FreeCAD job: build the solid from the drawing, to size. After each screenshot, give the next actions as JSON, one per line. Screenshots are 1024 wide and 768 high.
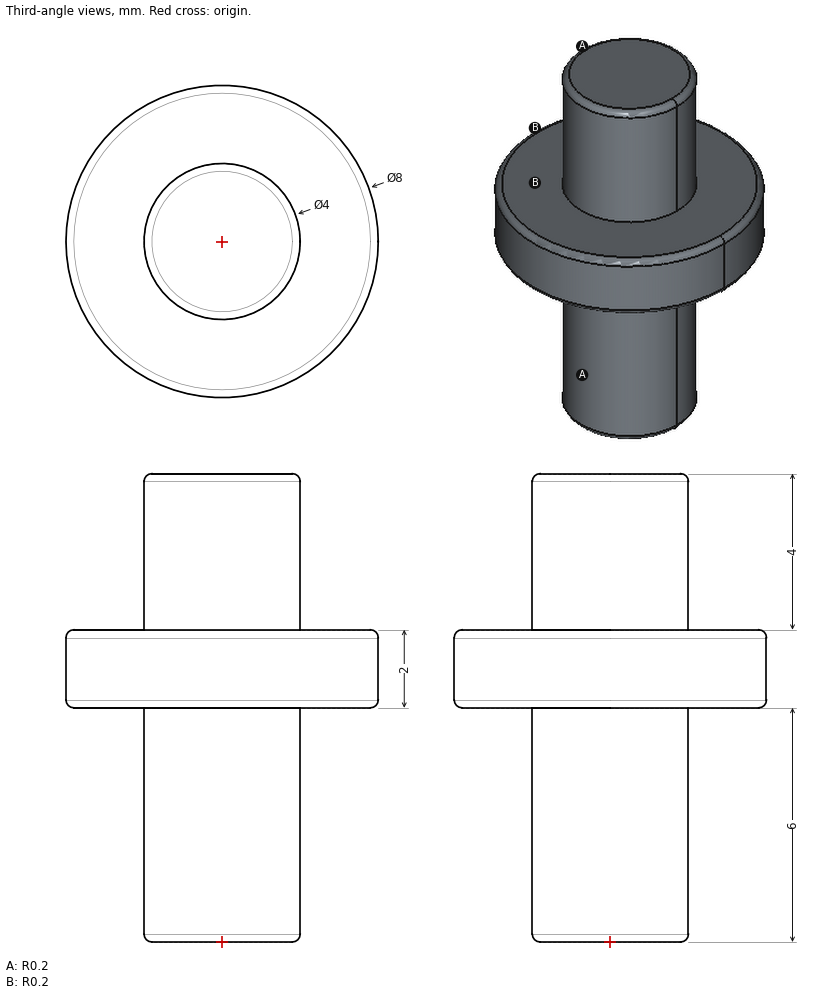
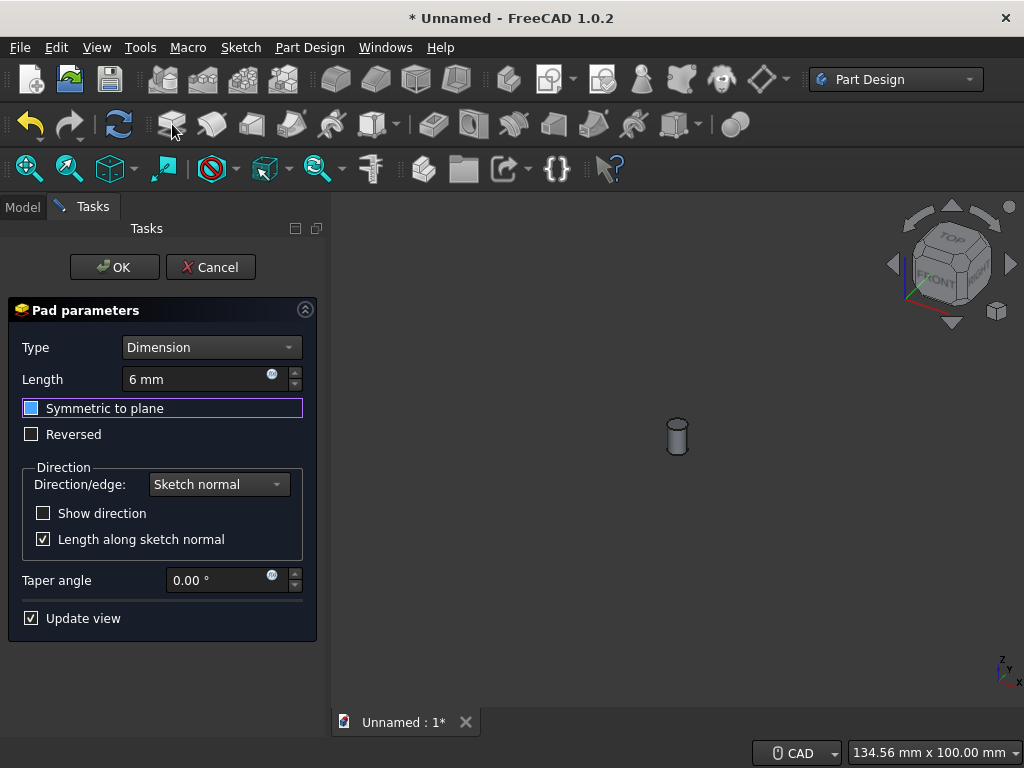
{"action": "left_click", "coordinate": [115, 267]}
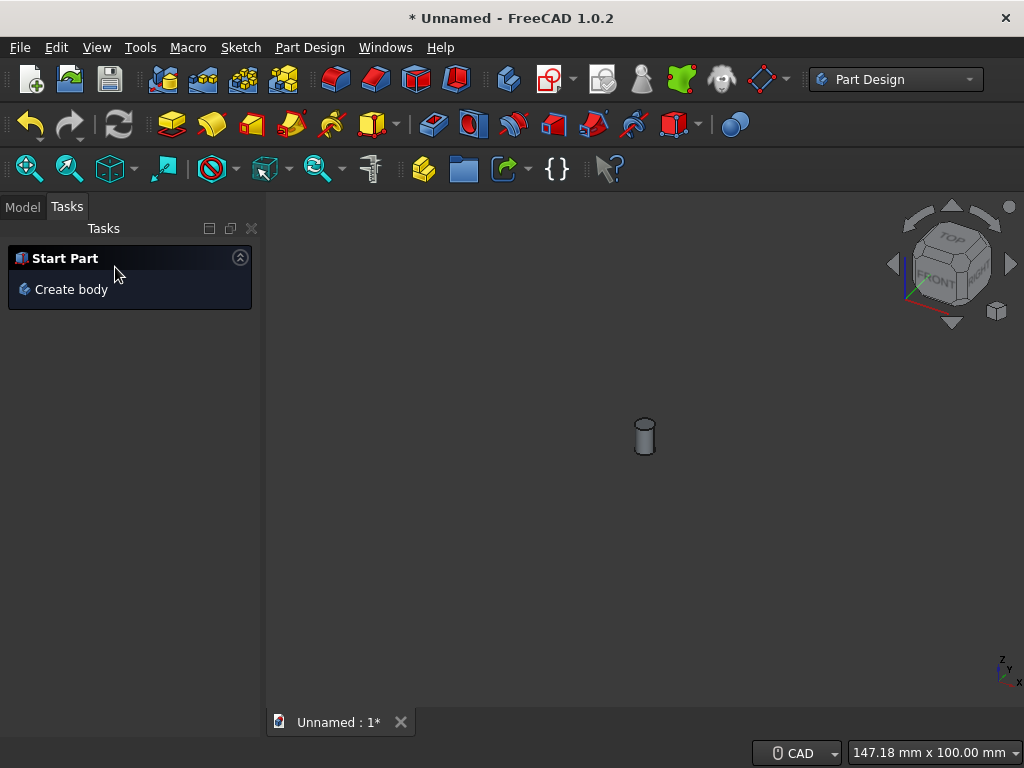
{"action": "left_click", "coordinate": [30, 170]}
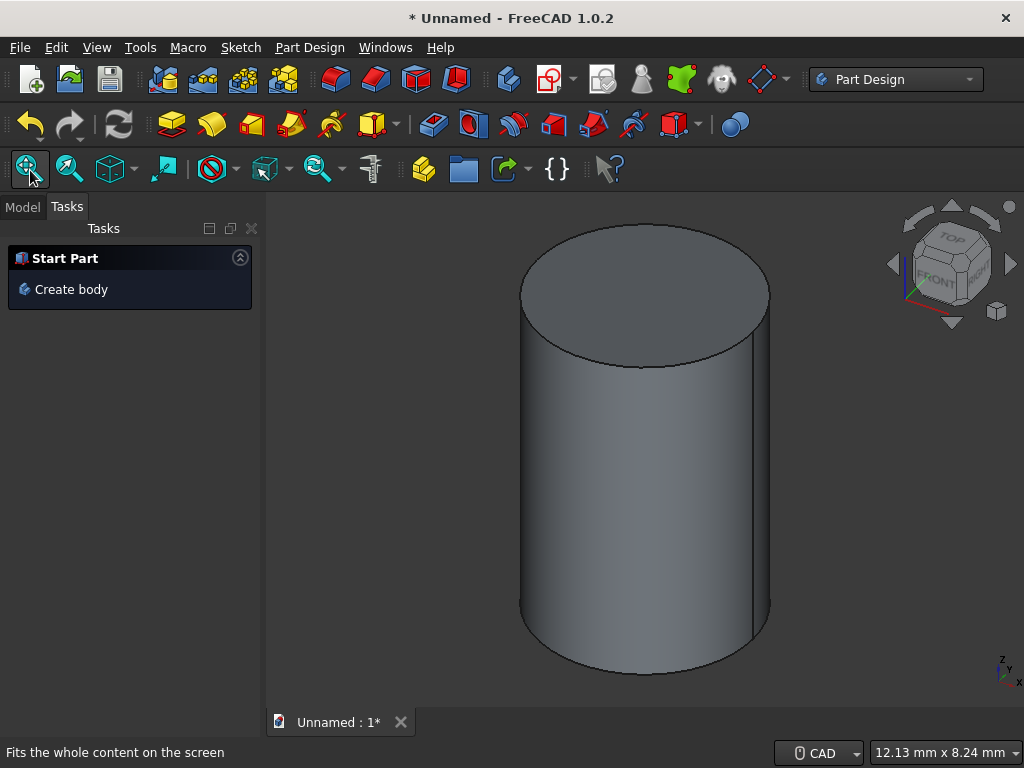
{"action": "left_click", "coordinate": [645, 295]}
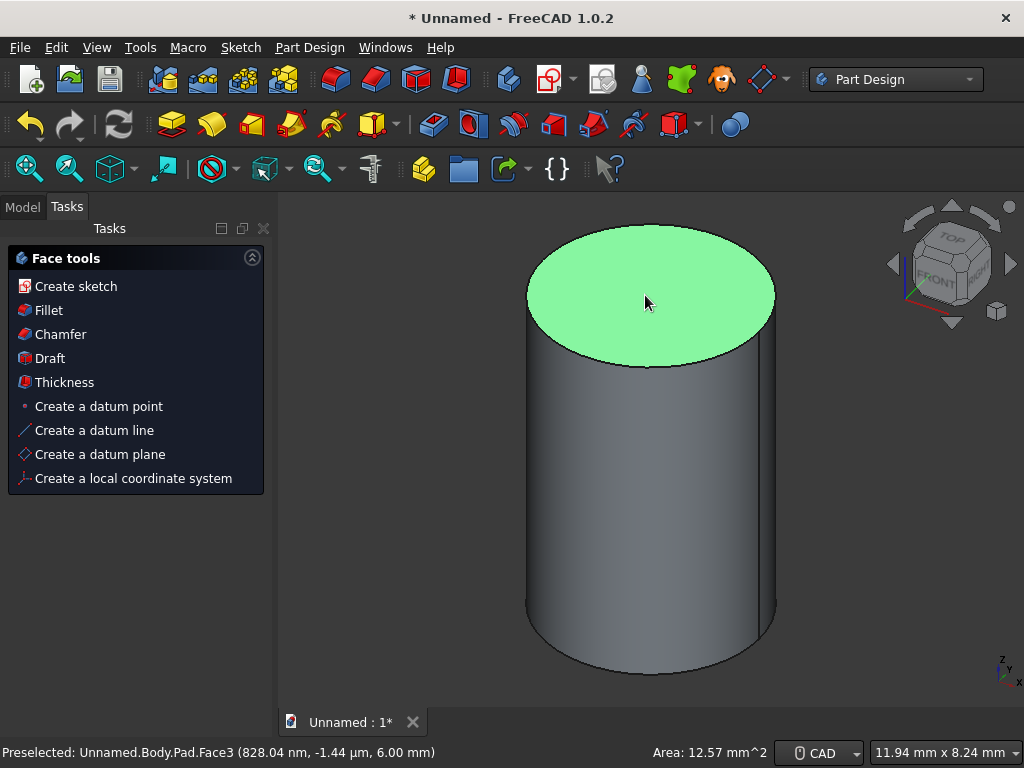
{"action": "left_click", "coordinate": [550, 80]}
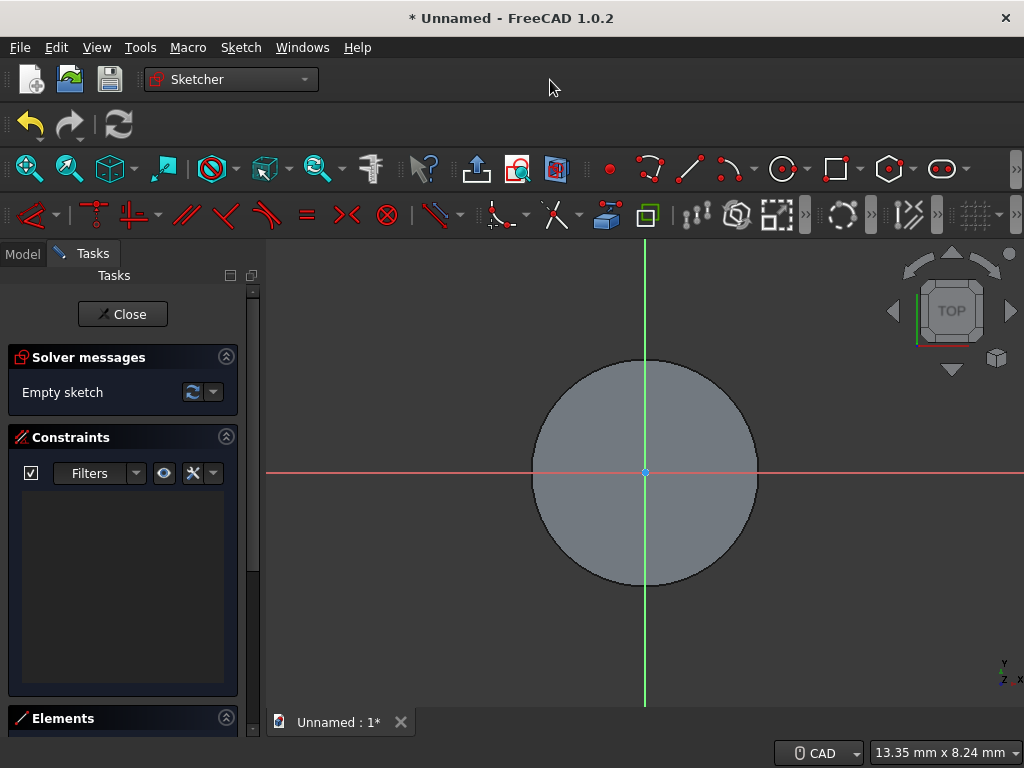
{"action": "scroll", "coordinate": [437, 473], "scroll_direction": "down", "scroll_amount": 2}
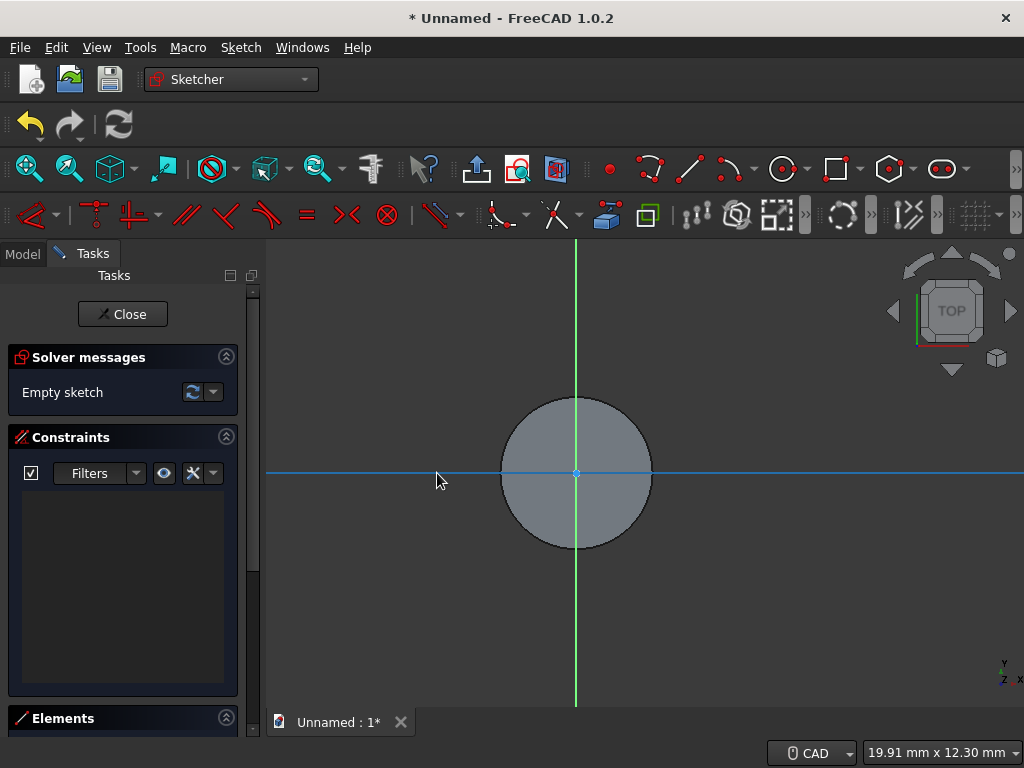
{"action": "left_click", "coordinate": [784, 170]}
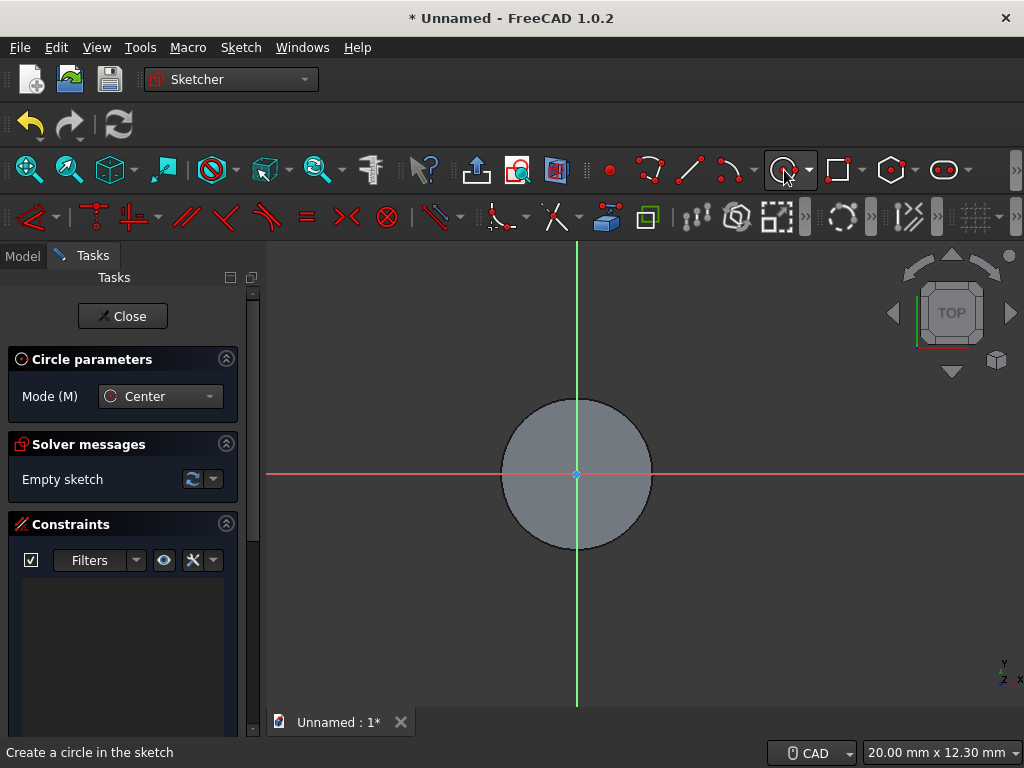
{"action": "left_click", "coordinate": [577, 474]}
{"action": "left_click", "coordinate": [684, 367]}
{"action": "key", "text": "Escape"}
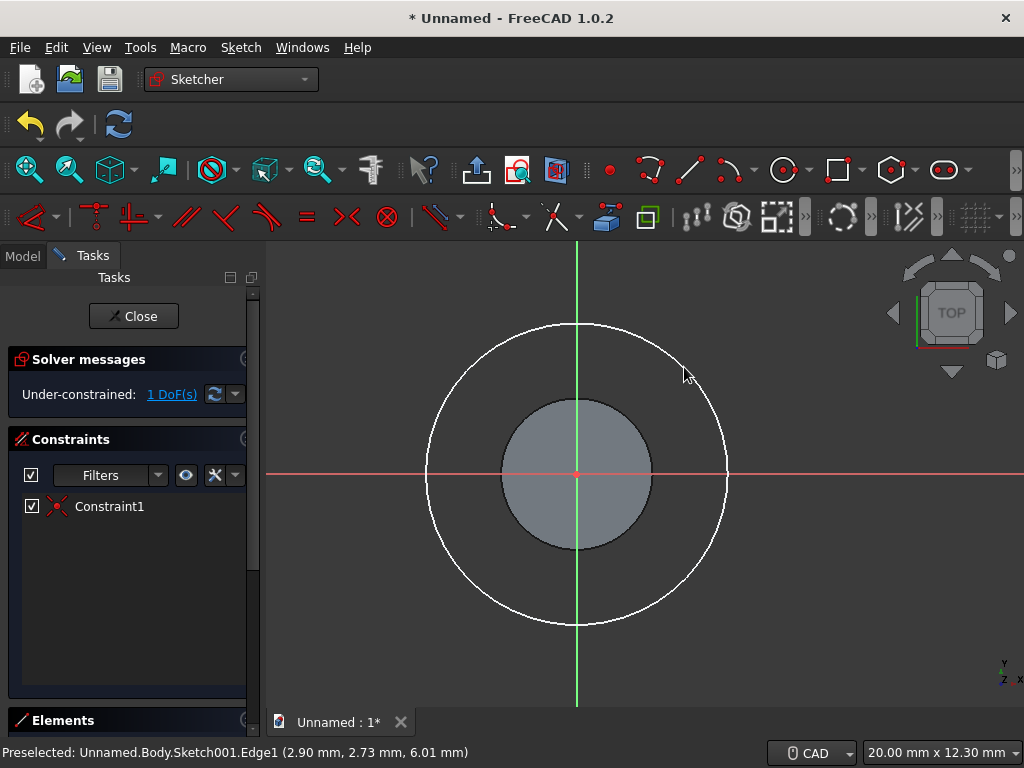
{"action": "left_click", "coordinate": [32, 218]}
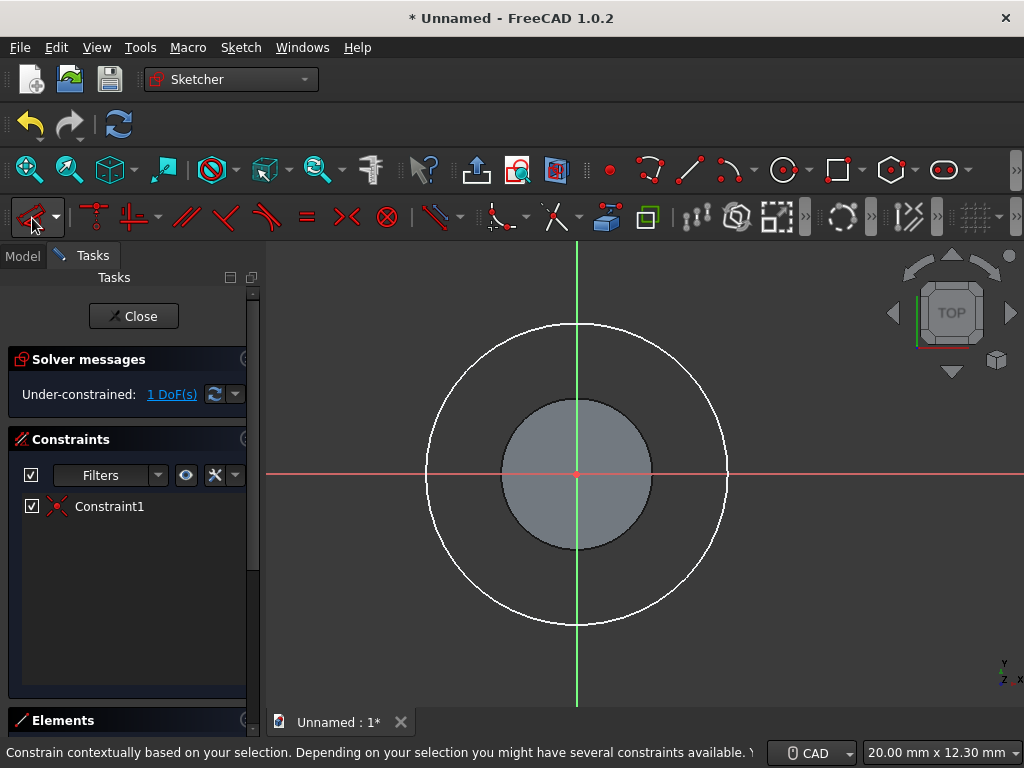
{"action": "left_click", "coordinate": [683, 367]}
{"action": "left_click", "coordinate": [706, 344]}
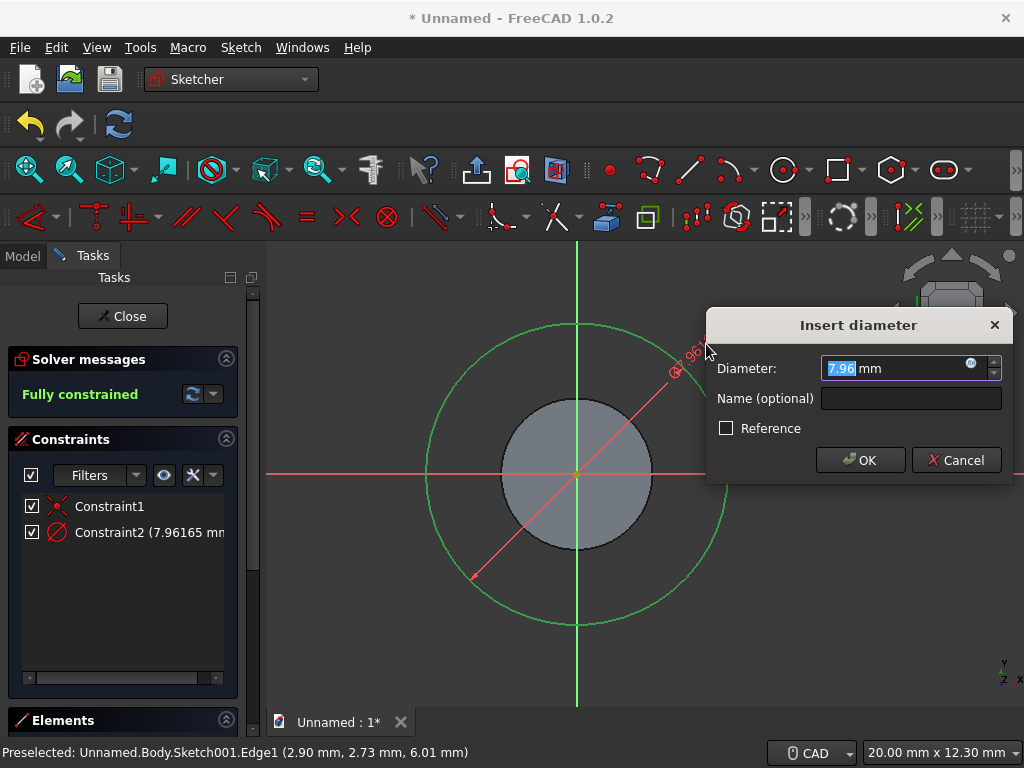
{"action": "type", "text": "8"}
{"action": "key", "text": "Return"}
{"action": "key", "text": "Escape"}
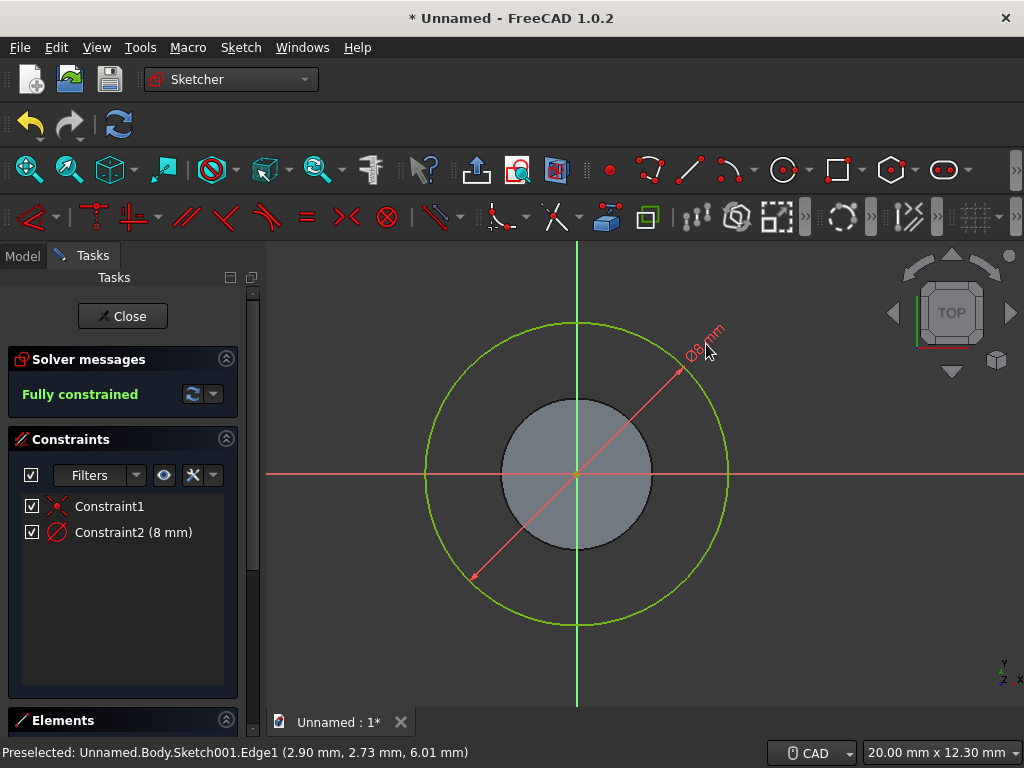
{"action": "left_click", "coordinate": [123, 316]}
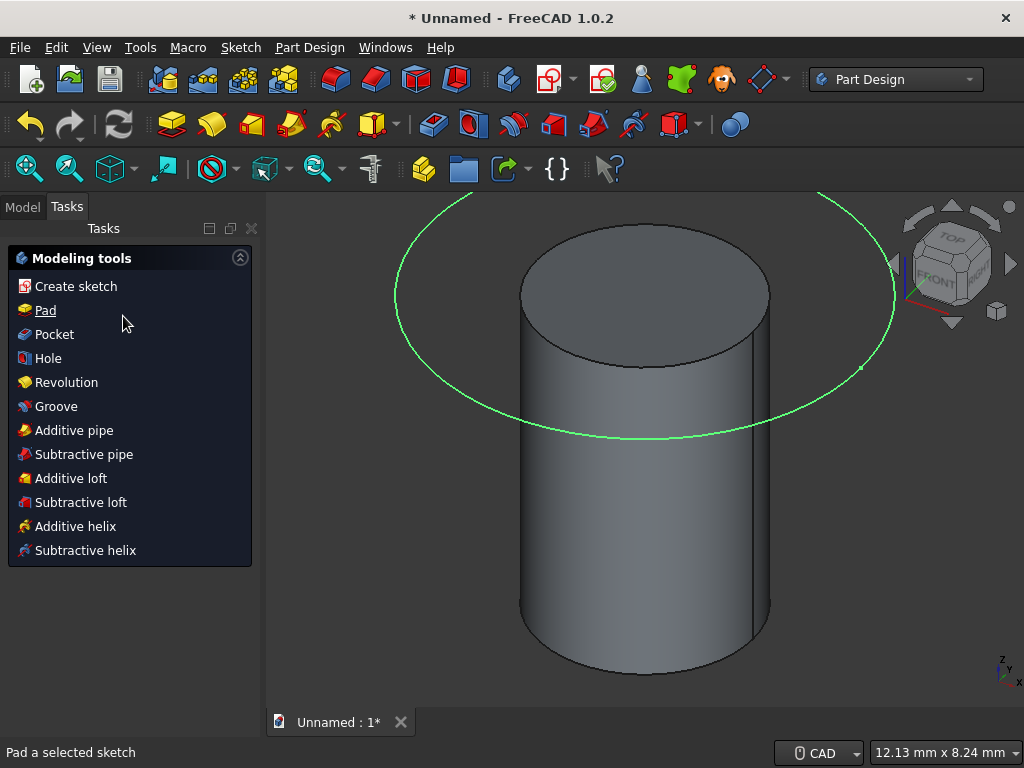
{"action": "left_click", "coordinate": [172, 124]}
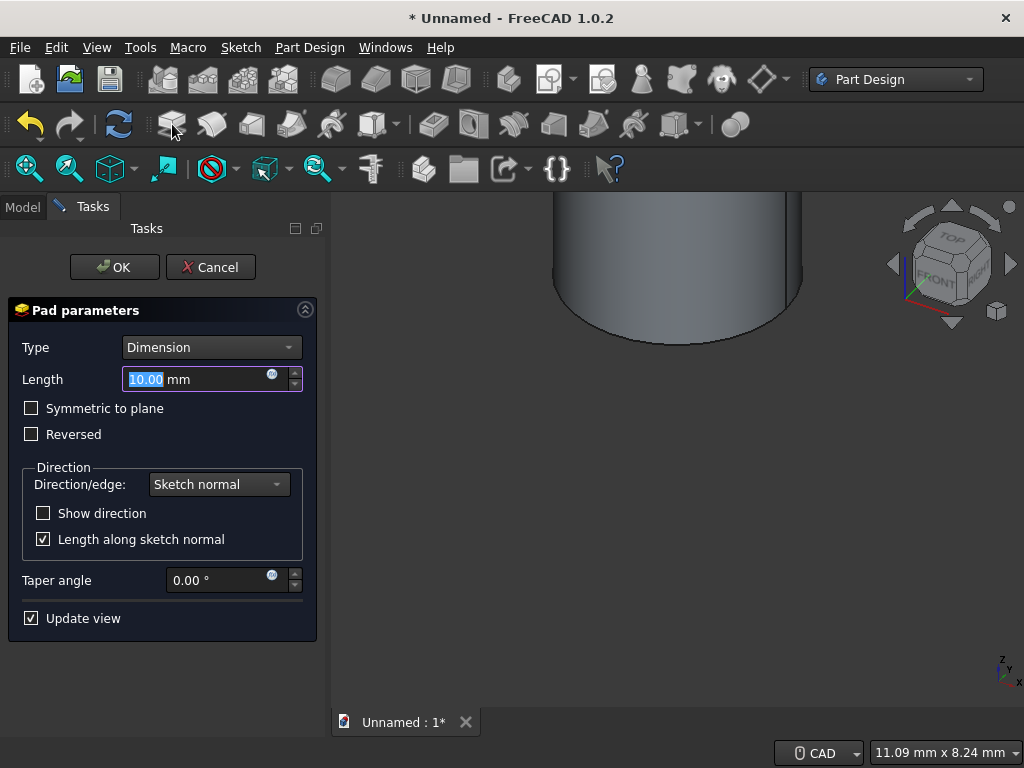
{"action": "type", "text": "2"}
{"action": "key", "text": "Tab"}